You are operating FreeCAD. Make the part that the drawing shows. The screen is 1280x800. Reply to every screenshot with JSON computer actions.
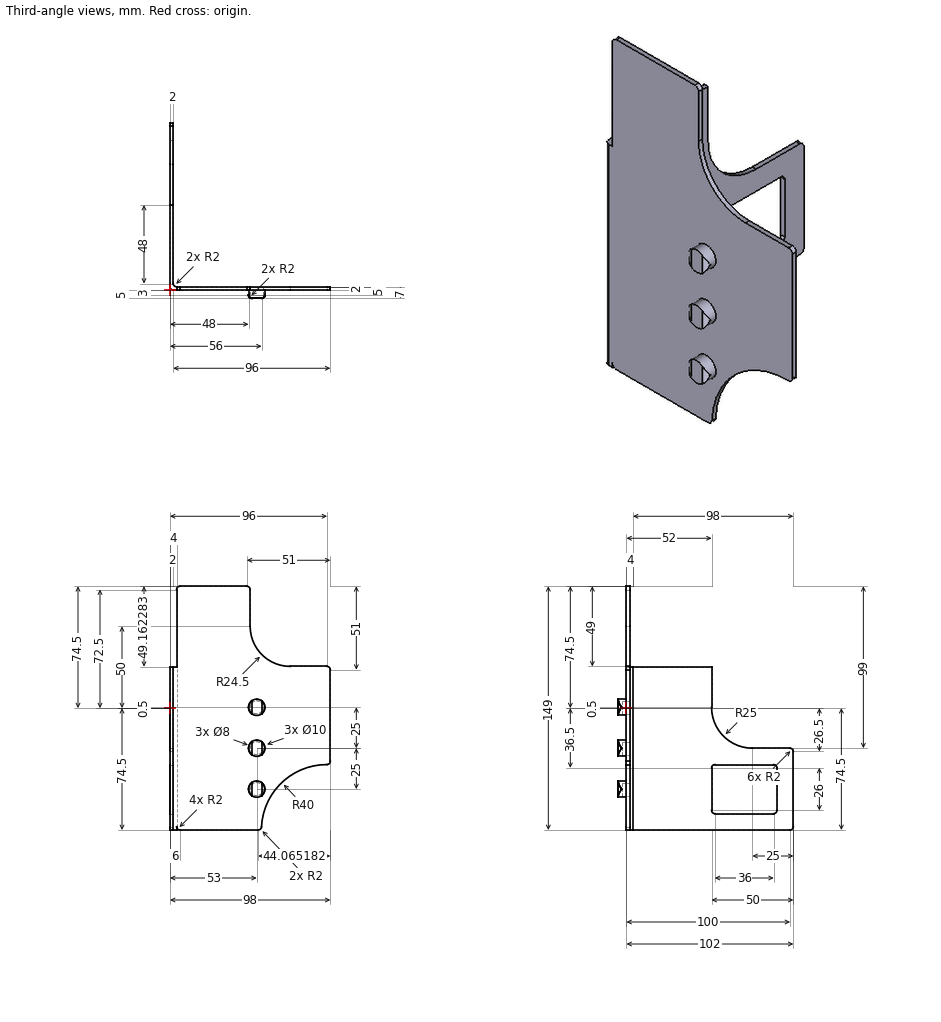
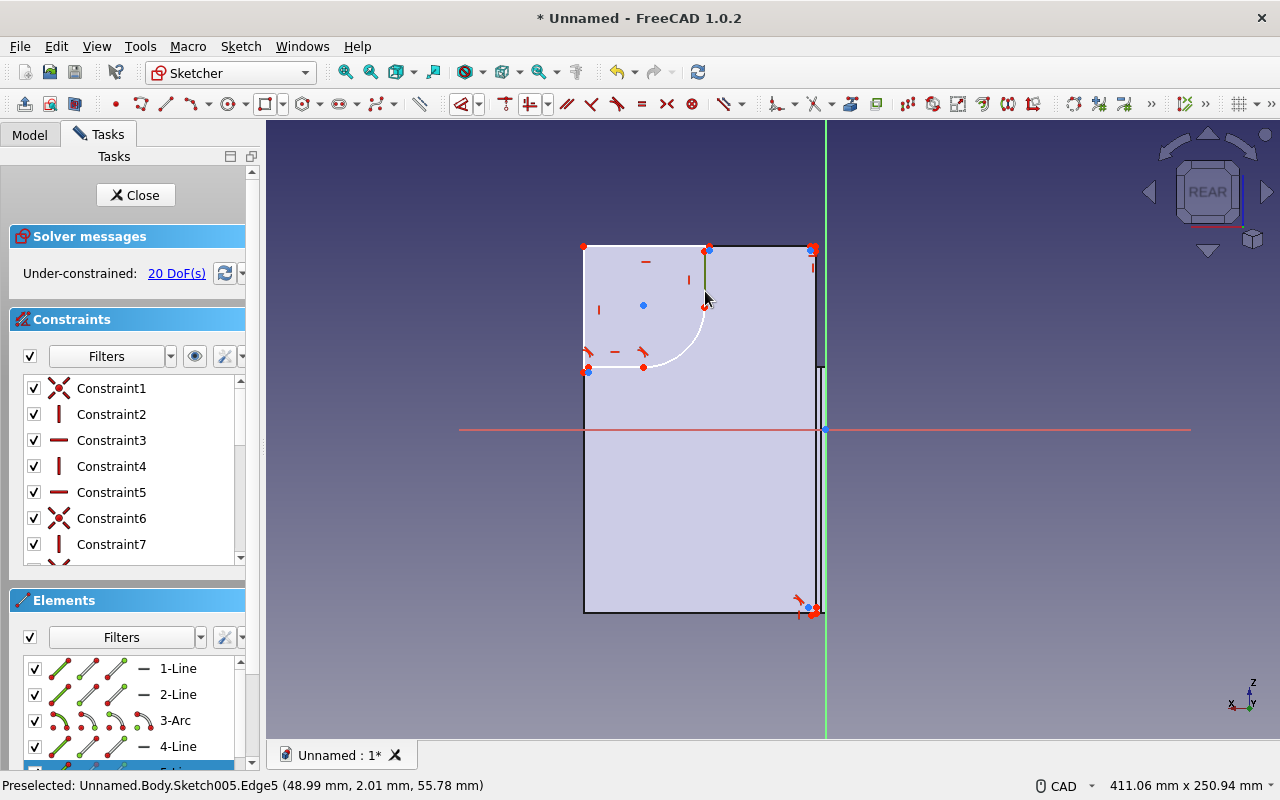
{"action": "left_click", "coordinate": [671, 361]}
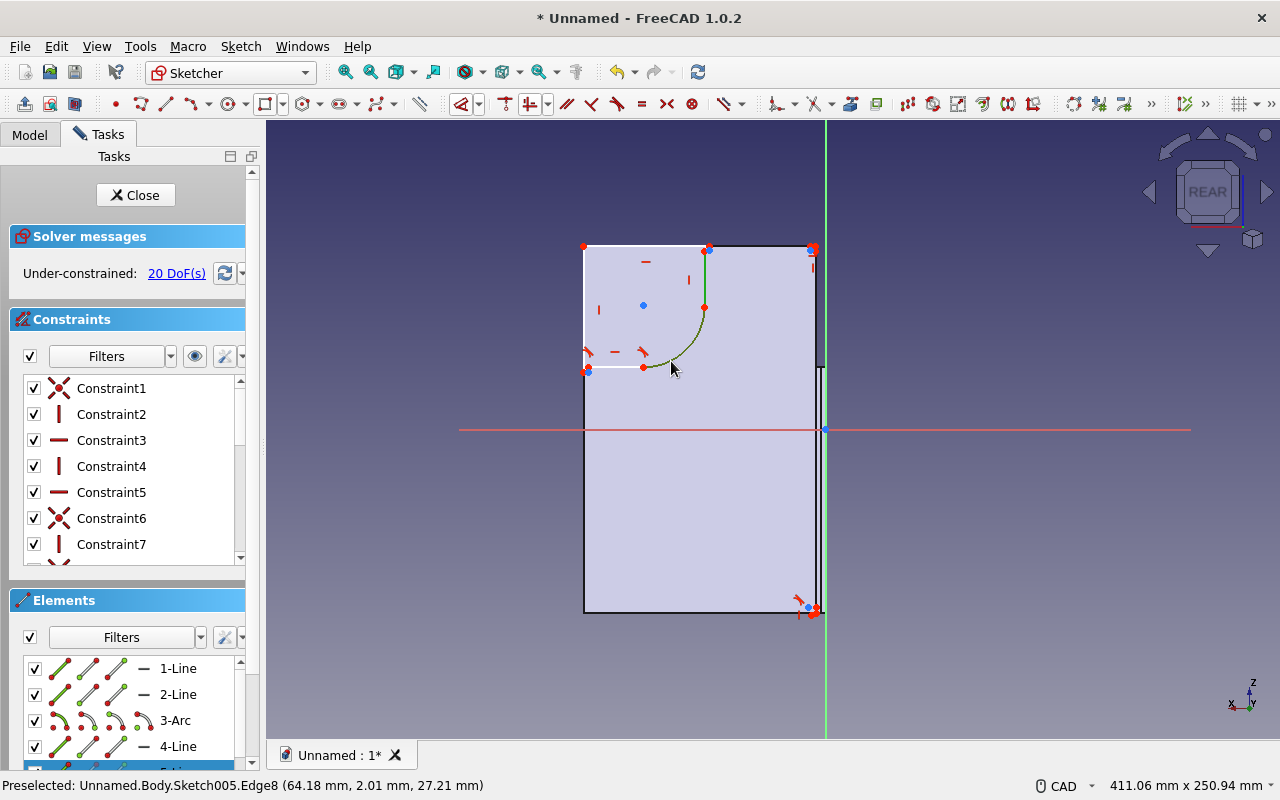
{"action": "key", "text": "t"}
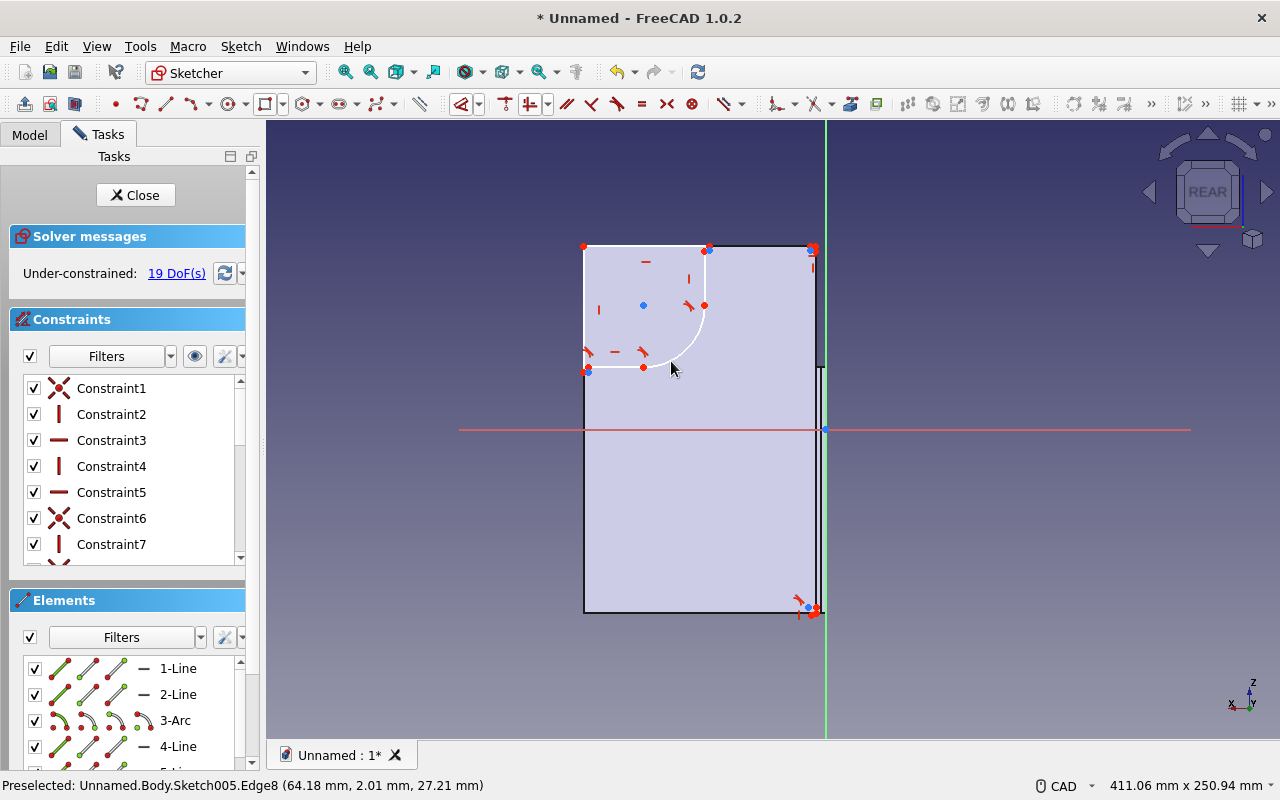
{"action": "left_click", "coordinate": [705, 289]}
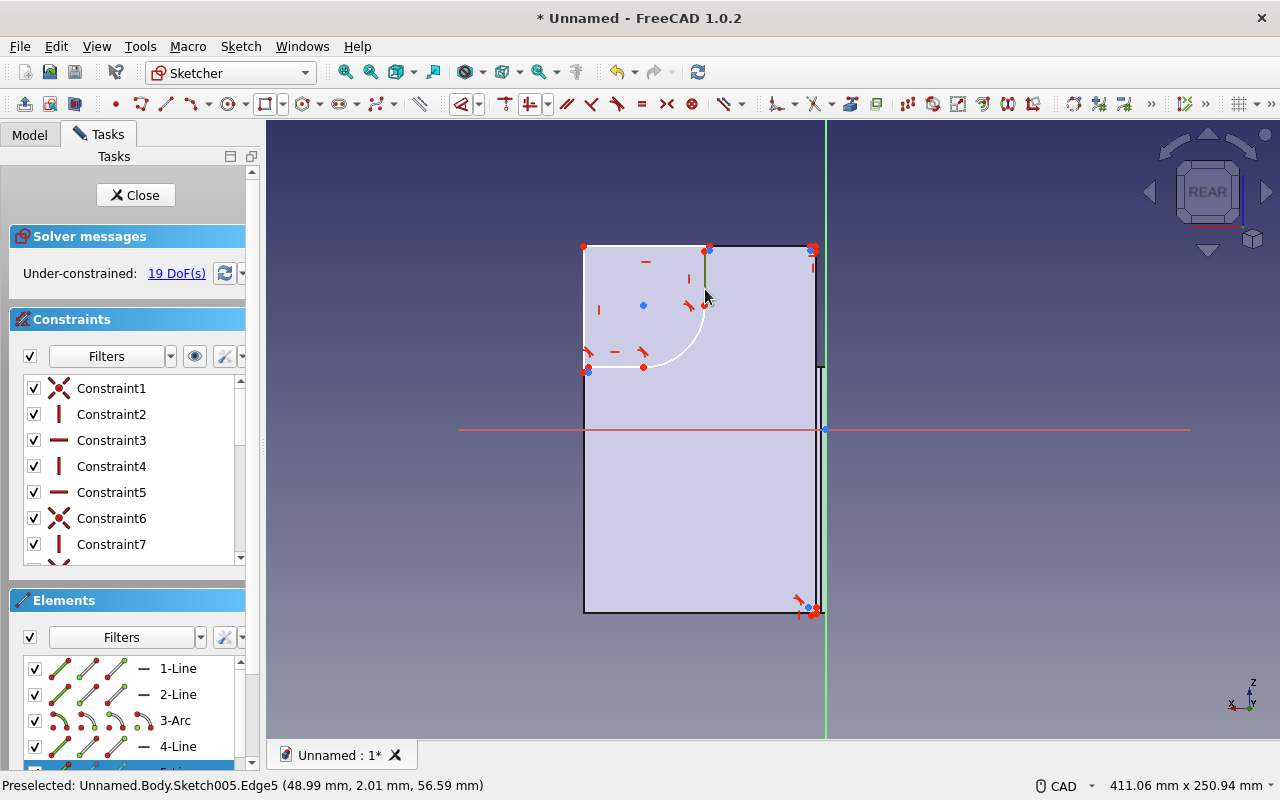
{"action": "scroll", "coordinate": [705, 249], "scroll_direction": "up", "scroll_amount": 9}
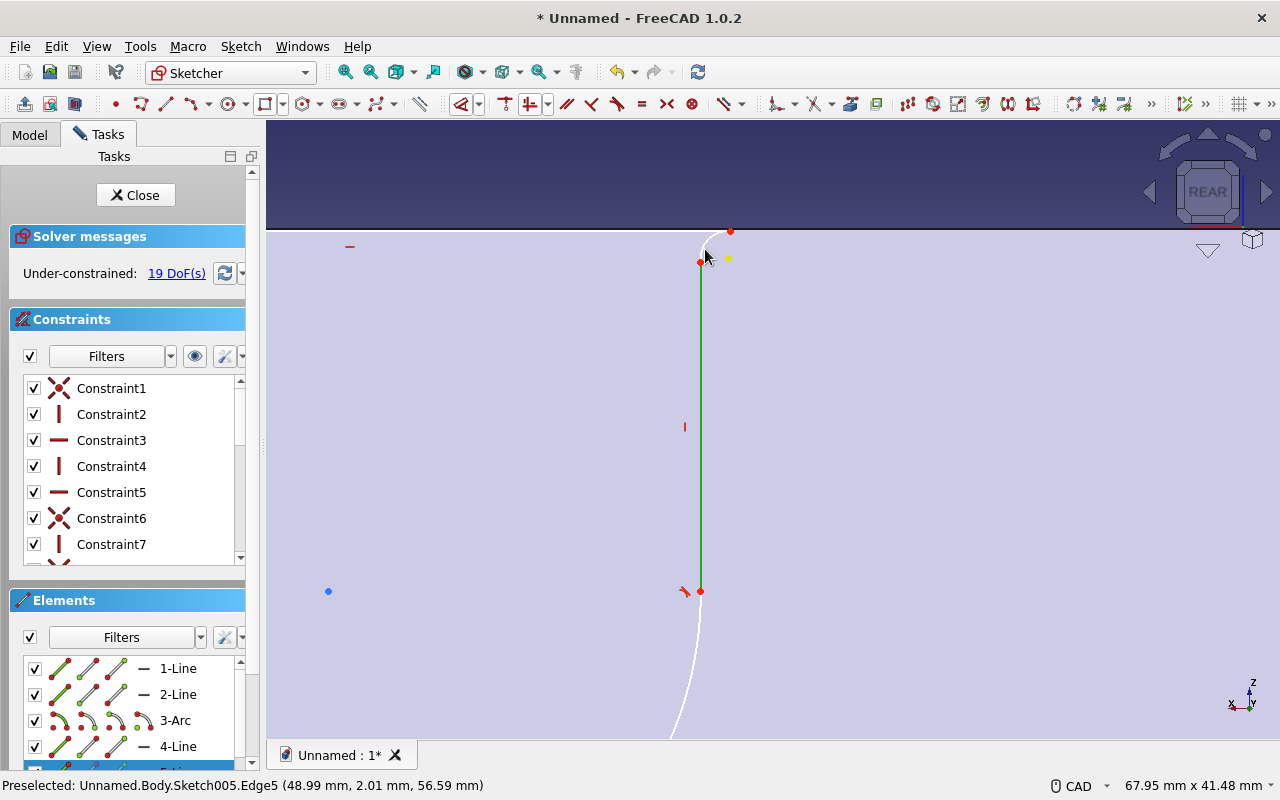
{"action": "left_click", "coordinate": [703, 248]}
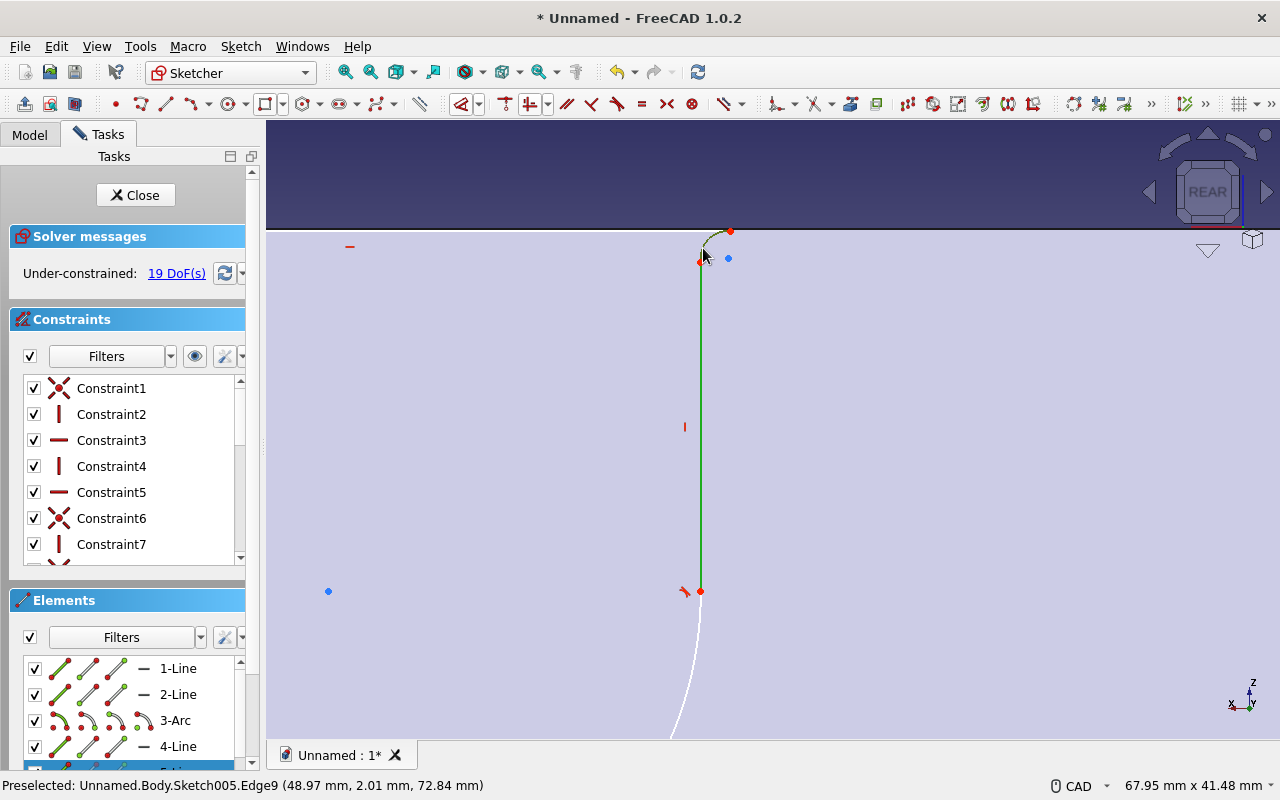
{"action": "key", "text": "t"}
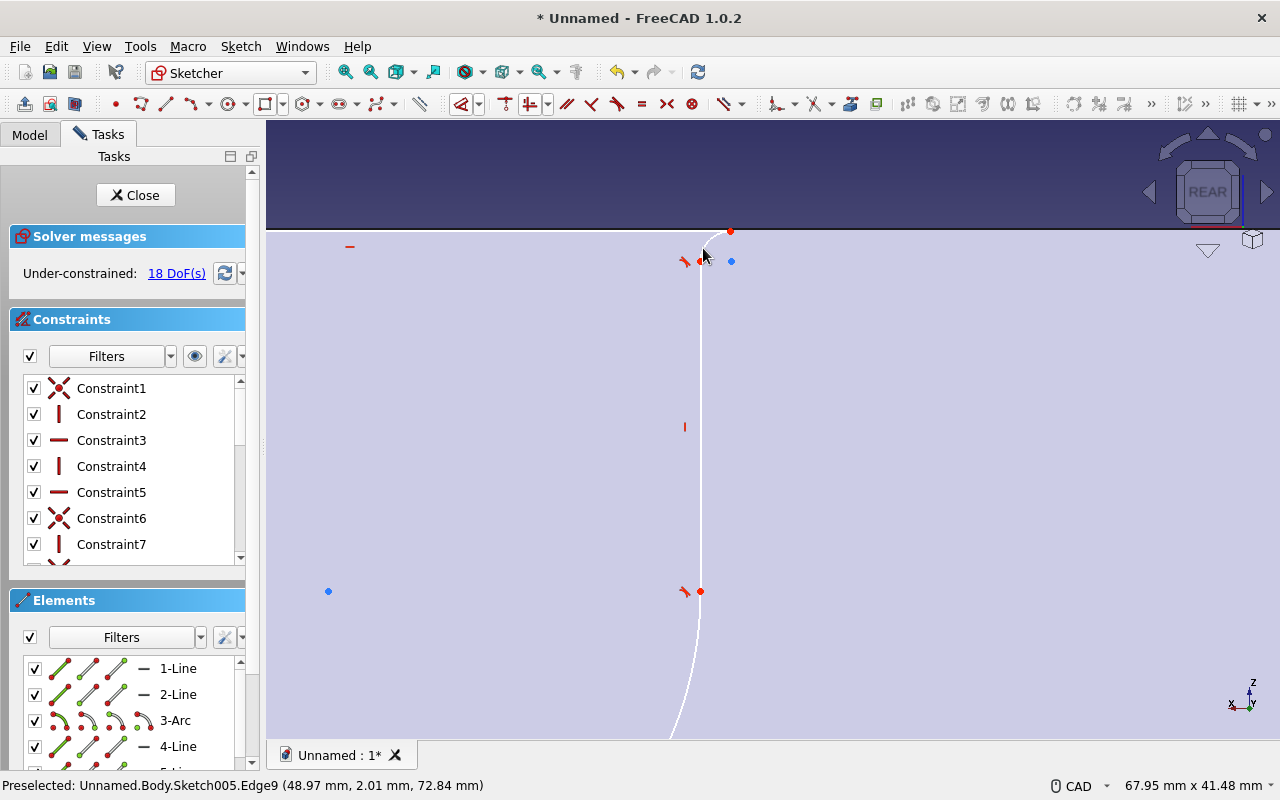
{"action": "scroll", "coordinate": [705, 249], "scroll_direction": "down", "scroll_amount": 9}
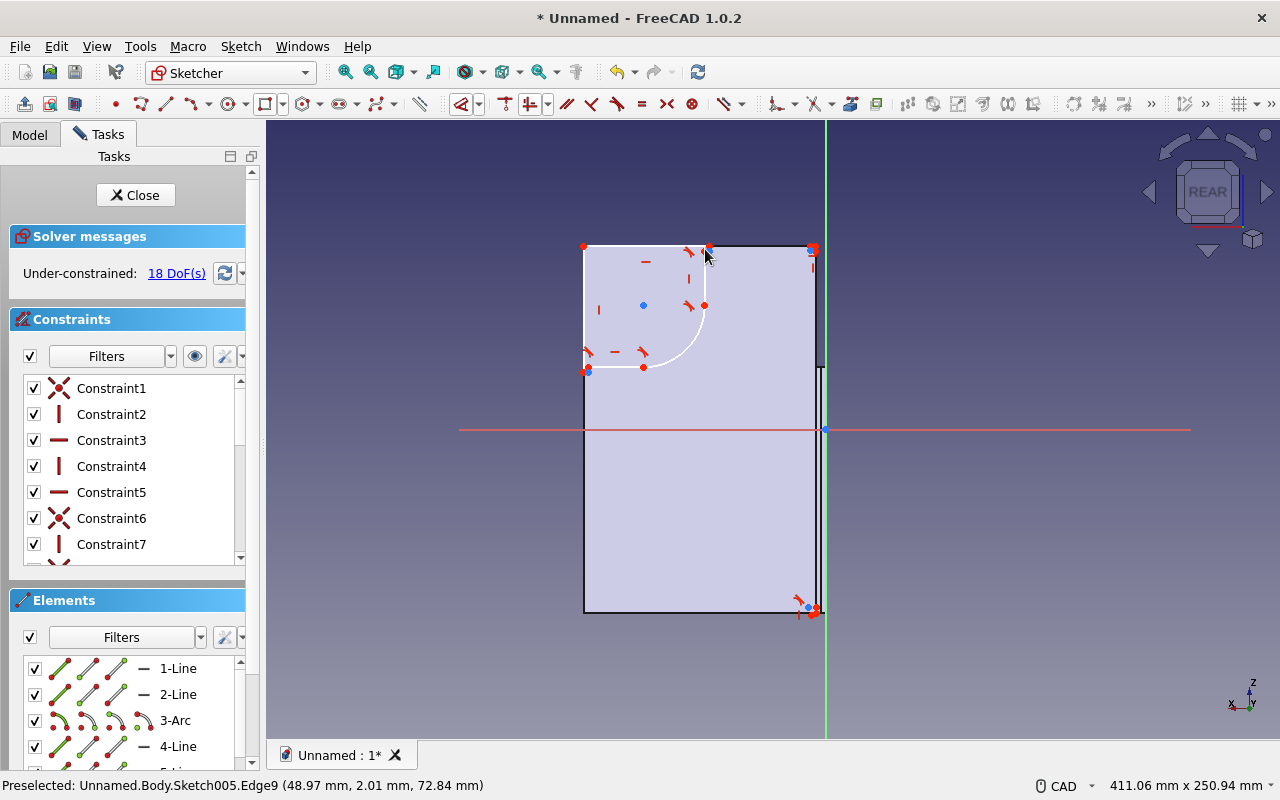
{"action": "left_click", "coordinate": [672, 246]}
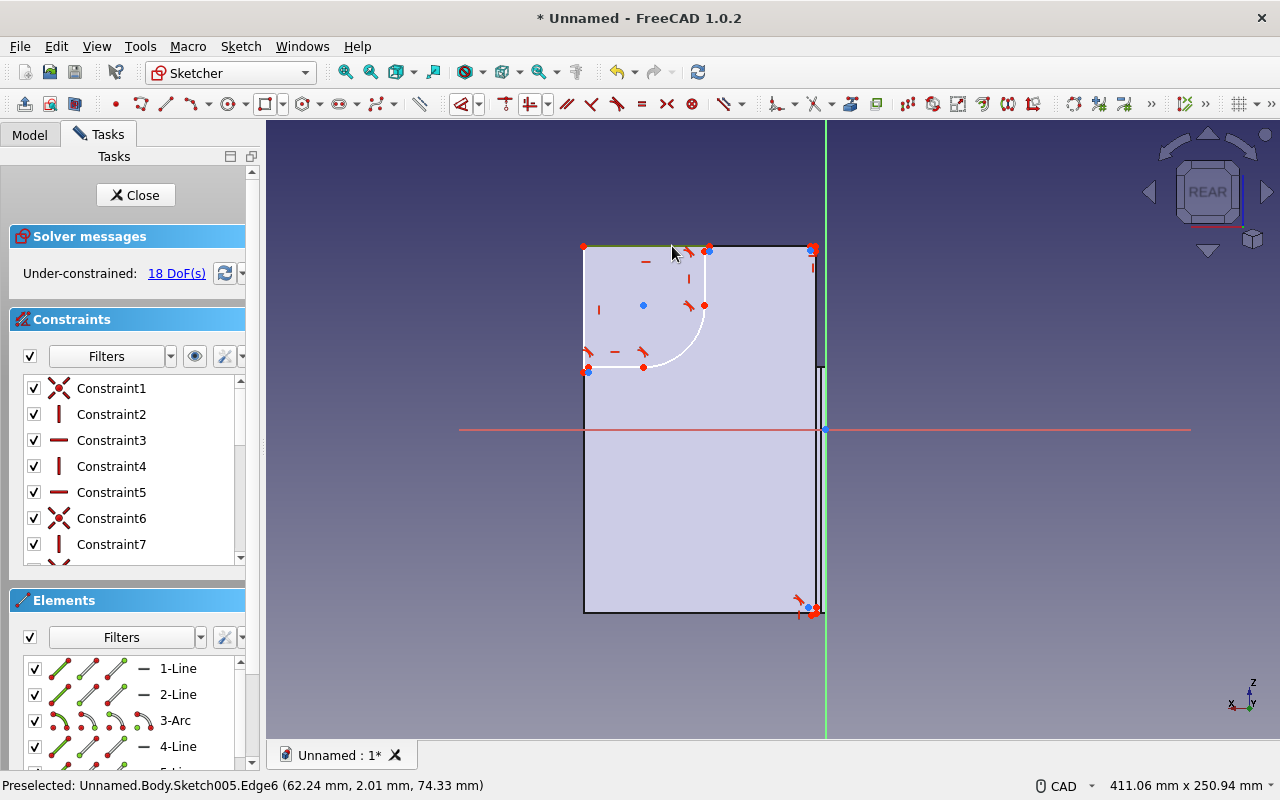
{"action": "scroll", "coordinate": [705, 249], "scroll_direction": "up", "scroll_amount": 9}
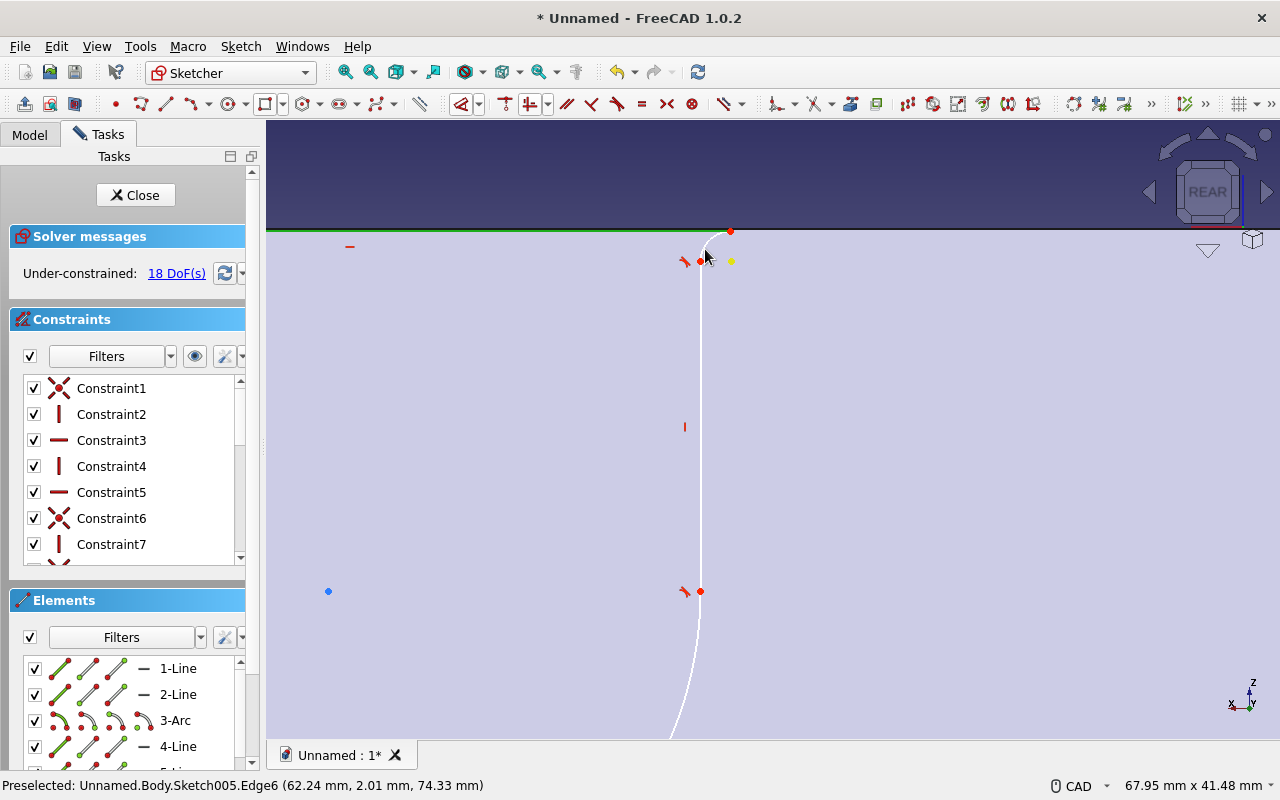
{"action": "left_click", "coordinate": [704, 248]}